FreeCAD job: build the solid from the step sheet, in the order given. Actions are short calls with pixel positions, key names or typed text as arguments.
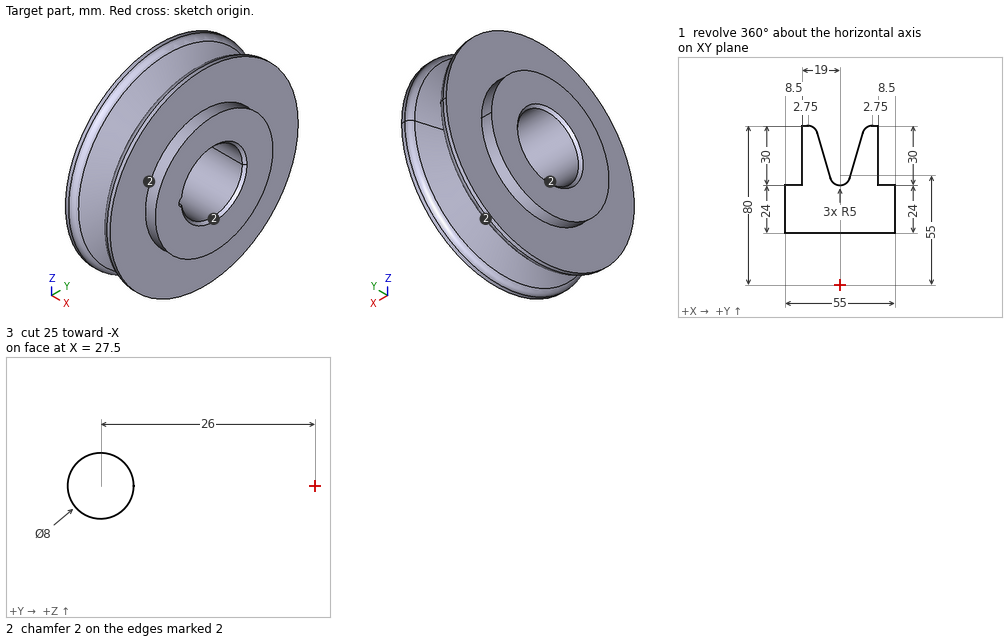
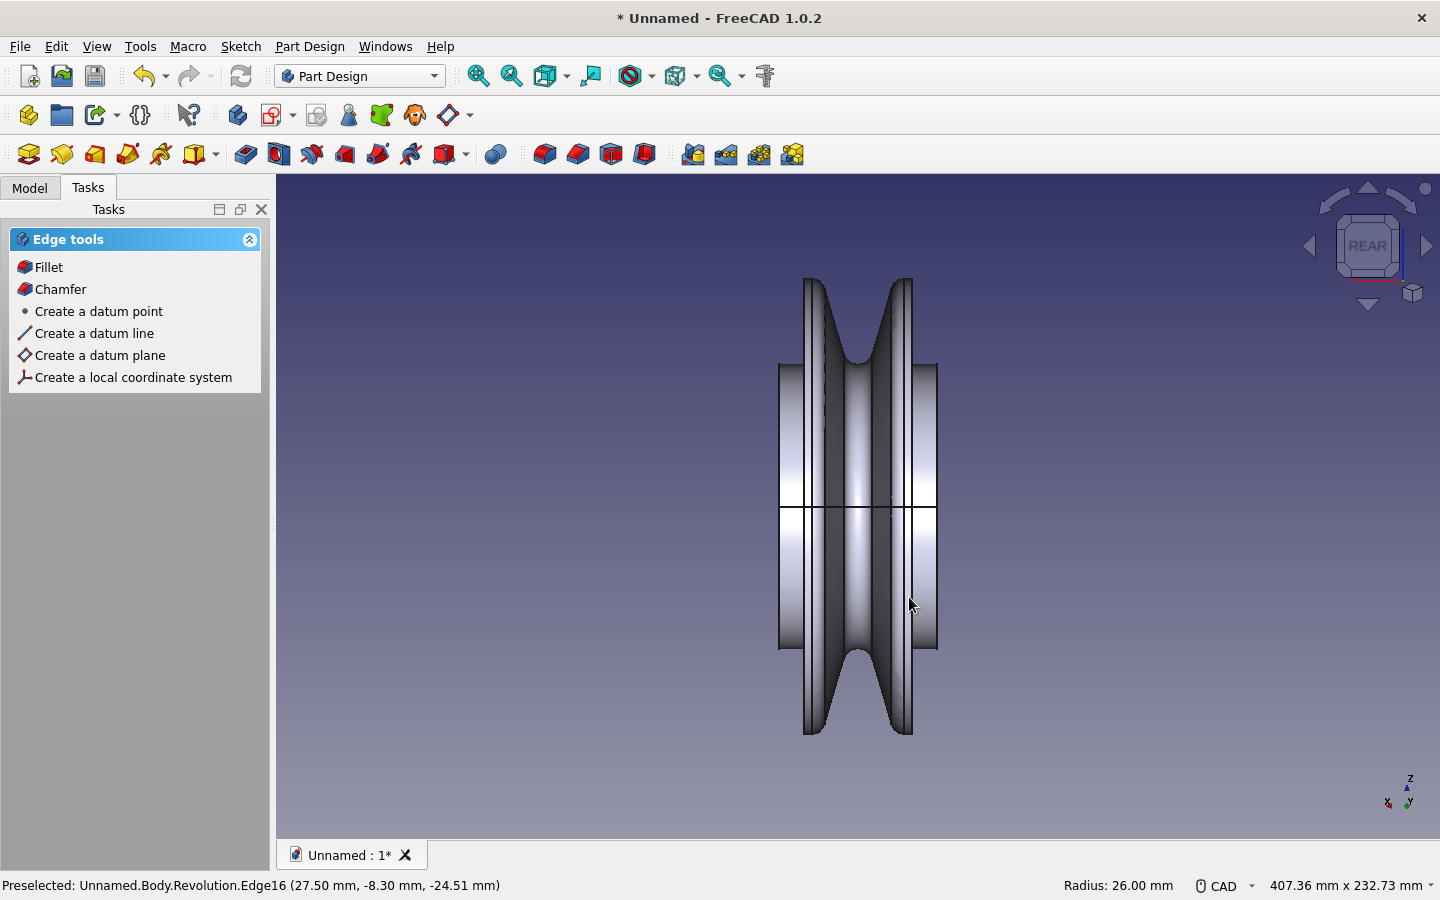
key(6)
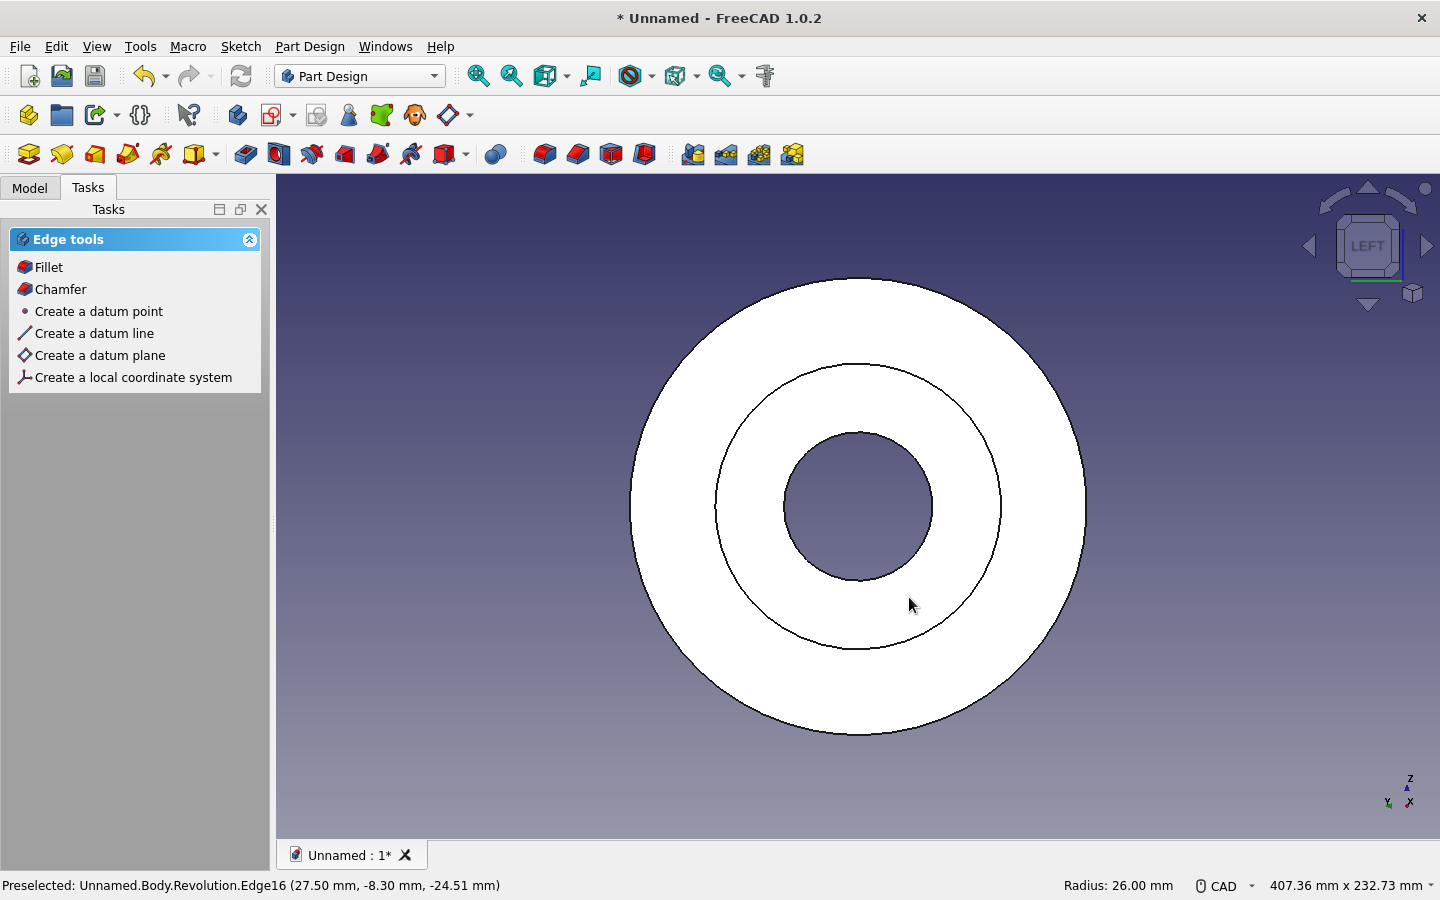
click(932, 505, ctrl)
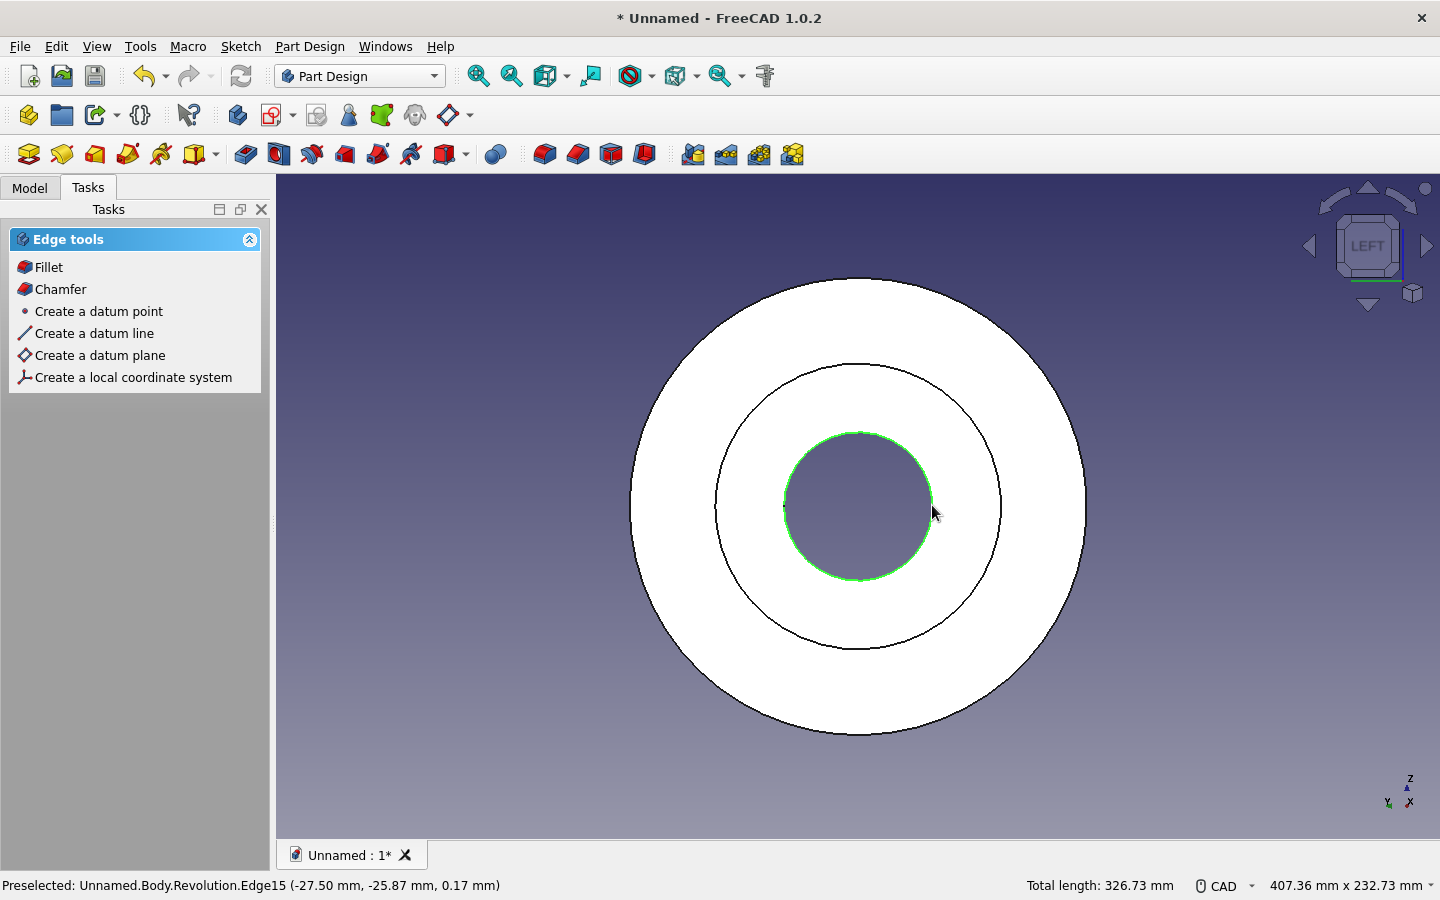
click(578, 154)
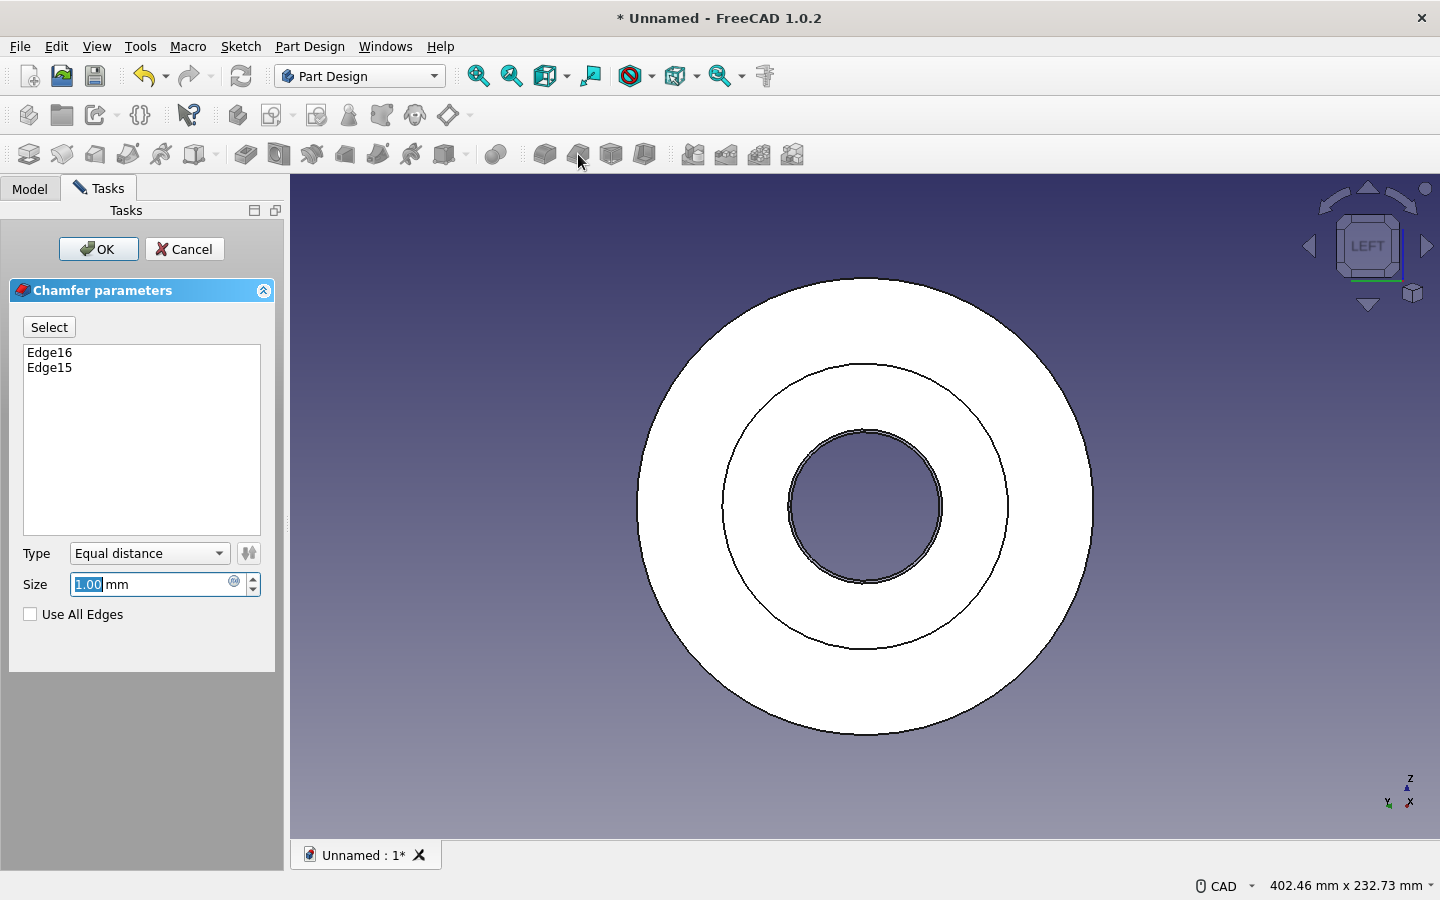
text(2)
key(Tab)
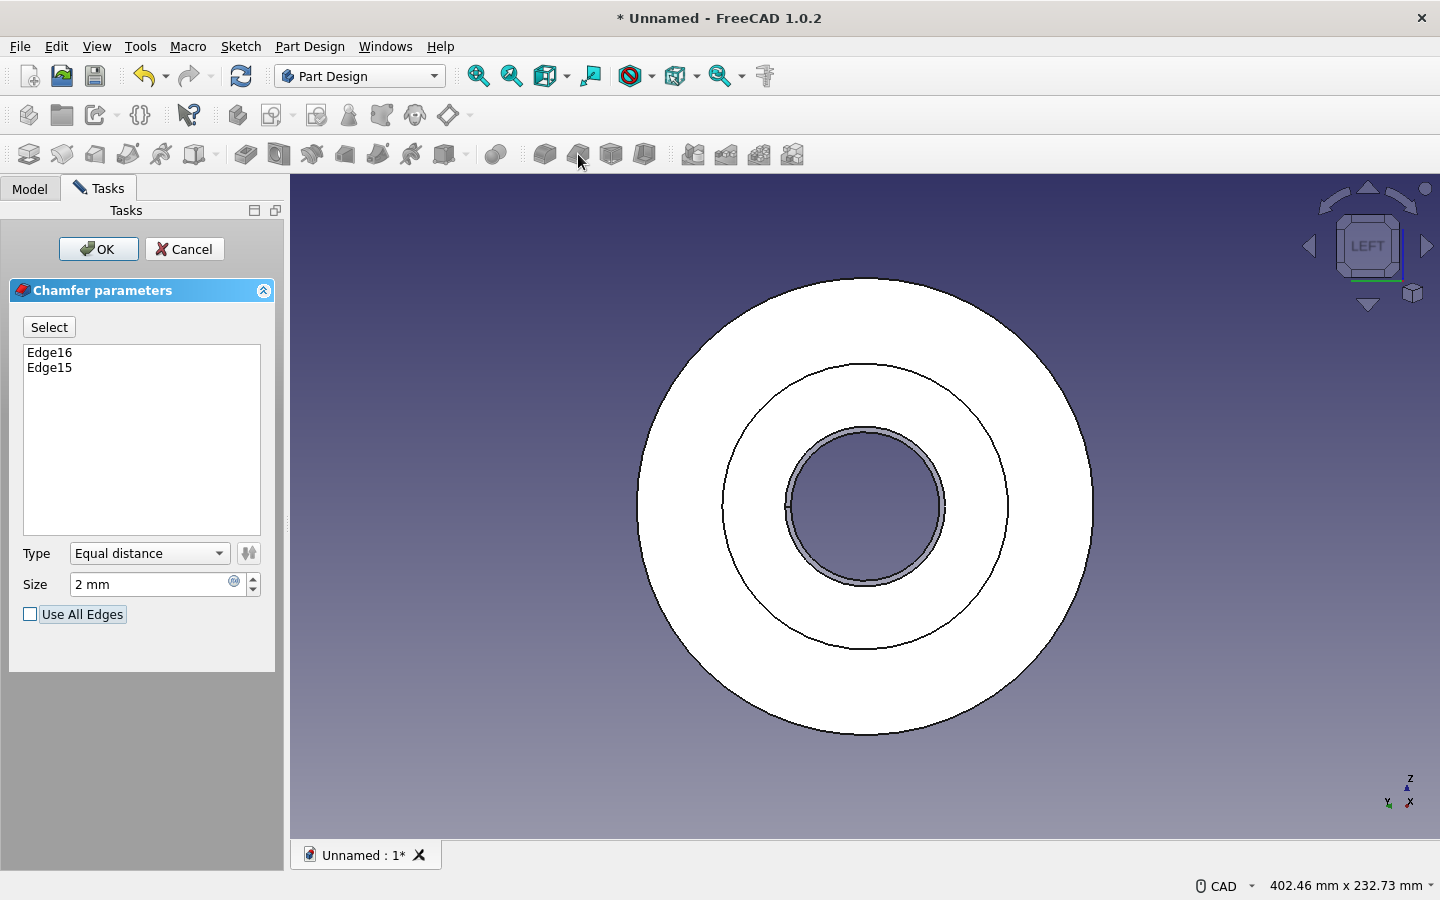
click(99, 249)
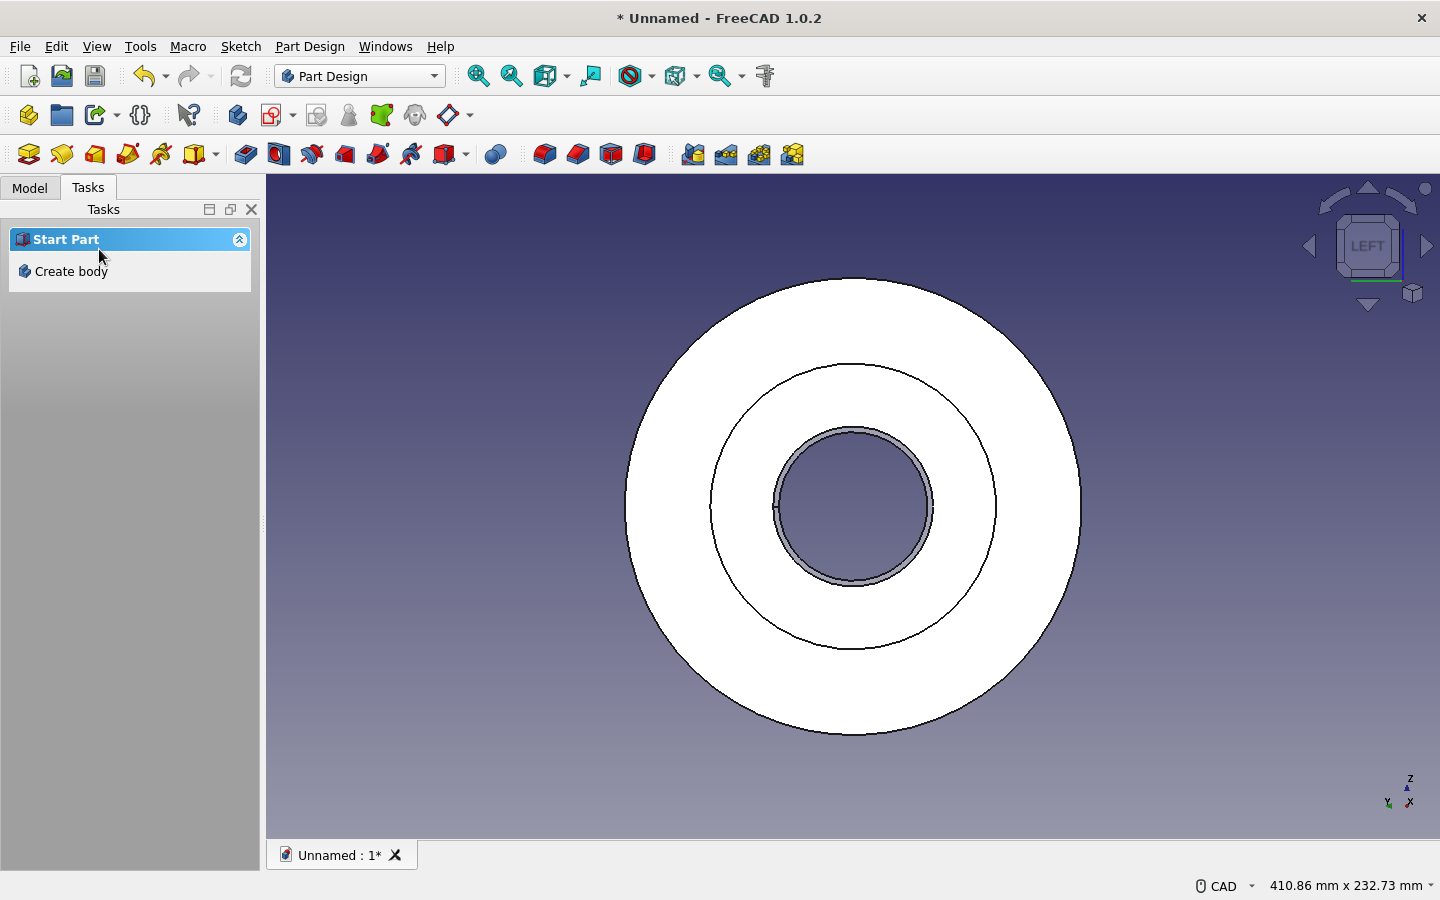
key(0)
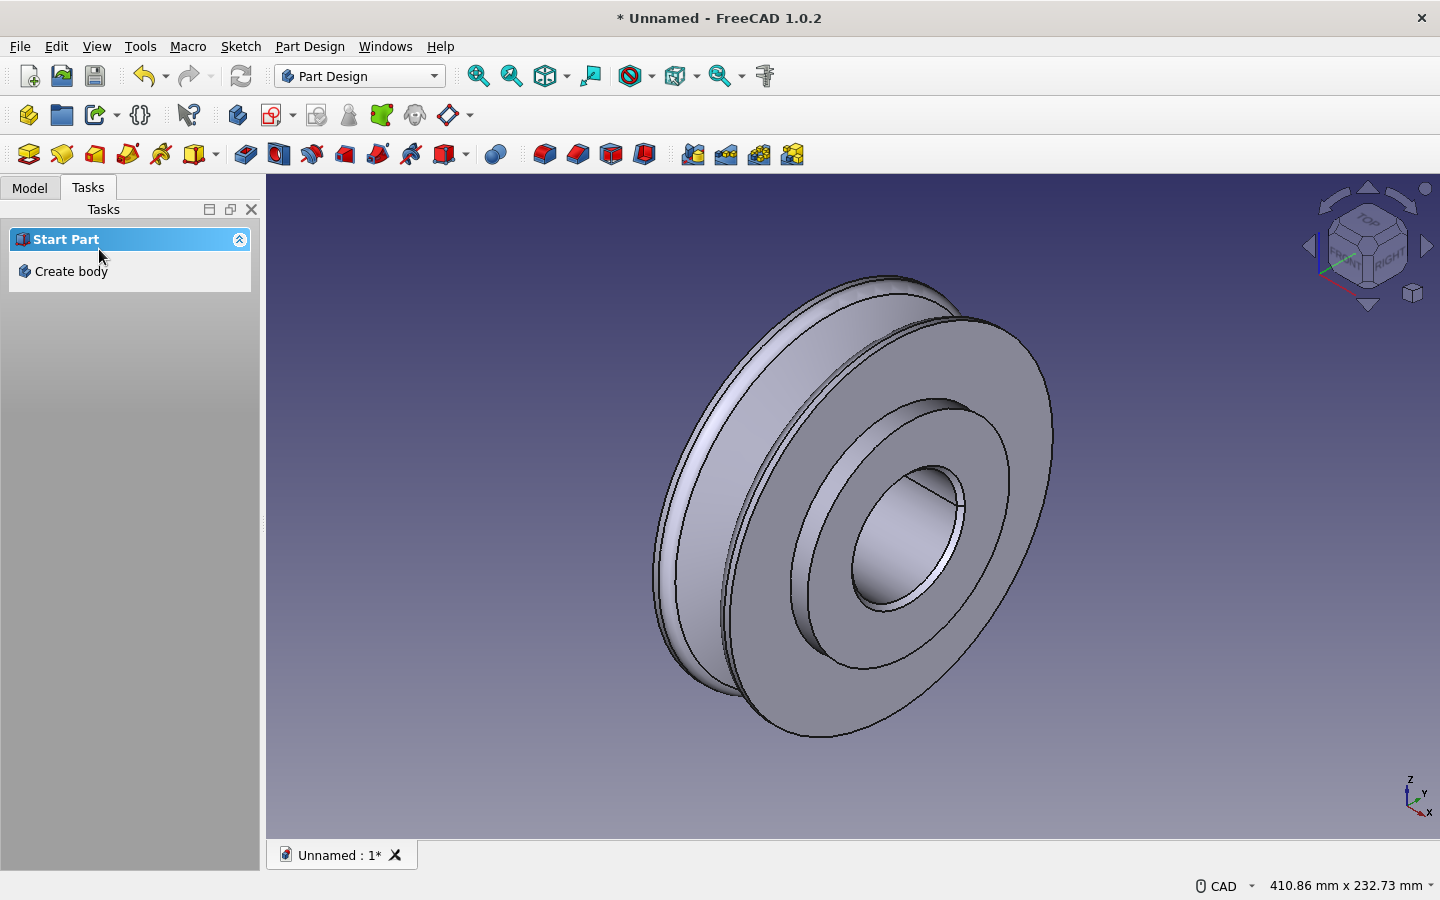
click(851, 638)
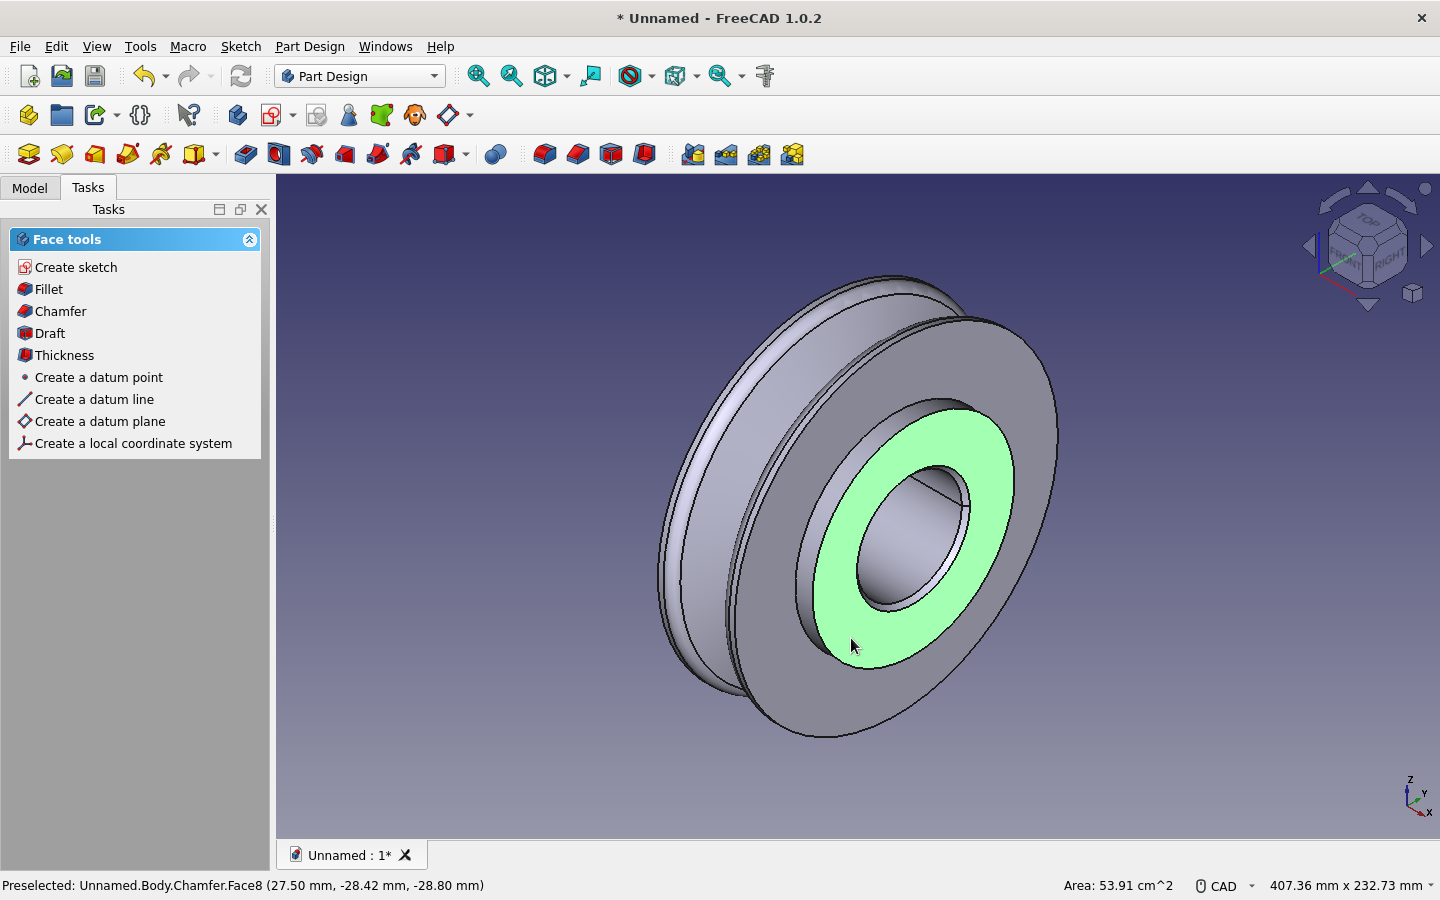
click(270, 116)